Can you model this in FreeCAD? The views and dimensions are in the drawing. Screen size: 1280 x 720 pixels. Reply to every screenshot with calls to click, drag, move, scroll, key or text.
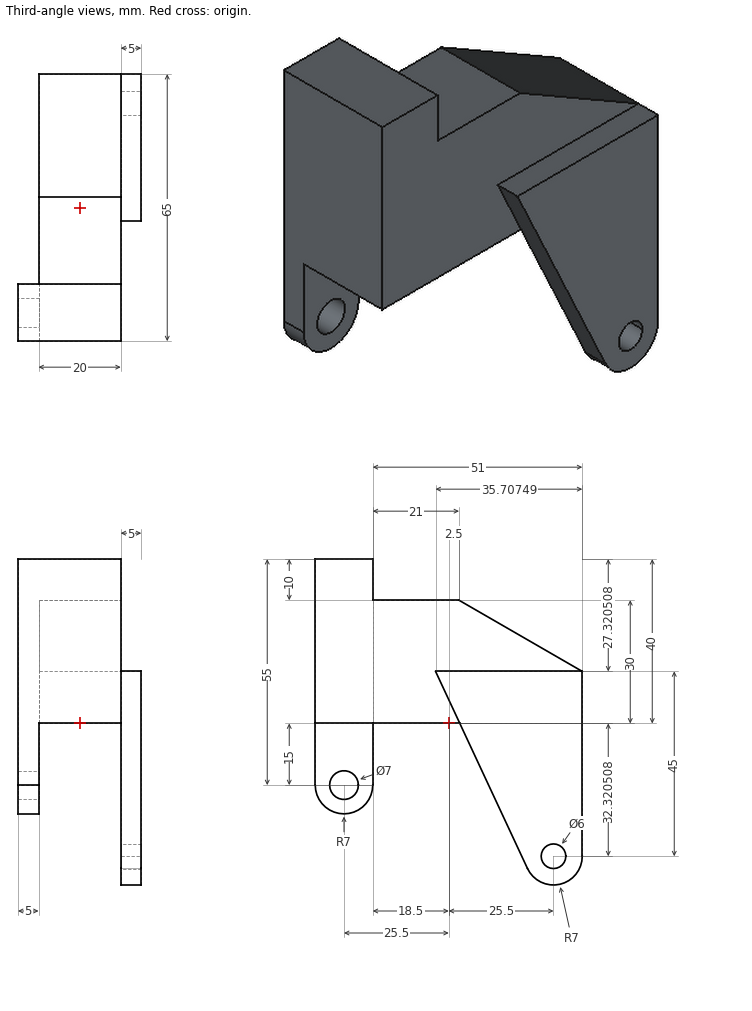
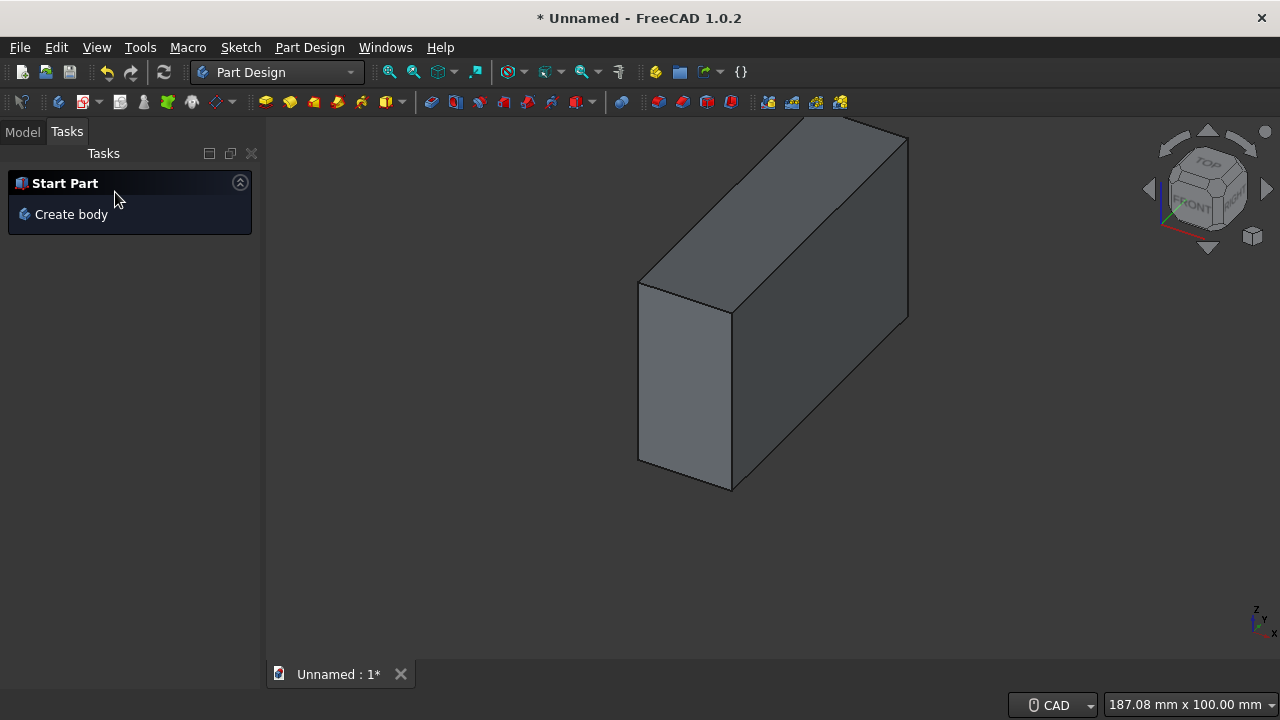
key(v)
key(f)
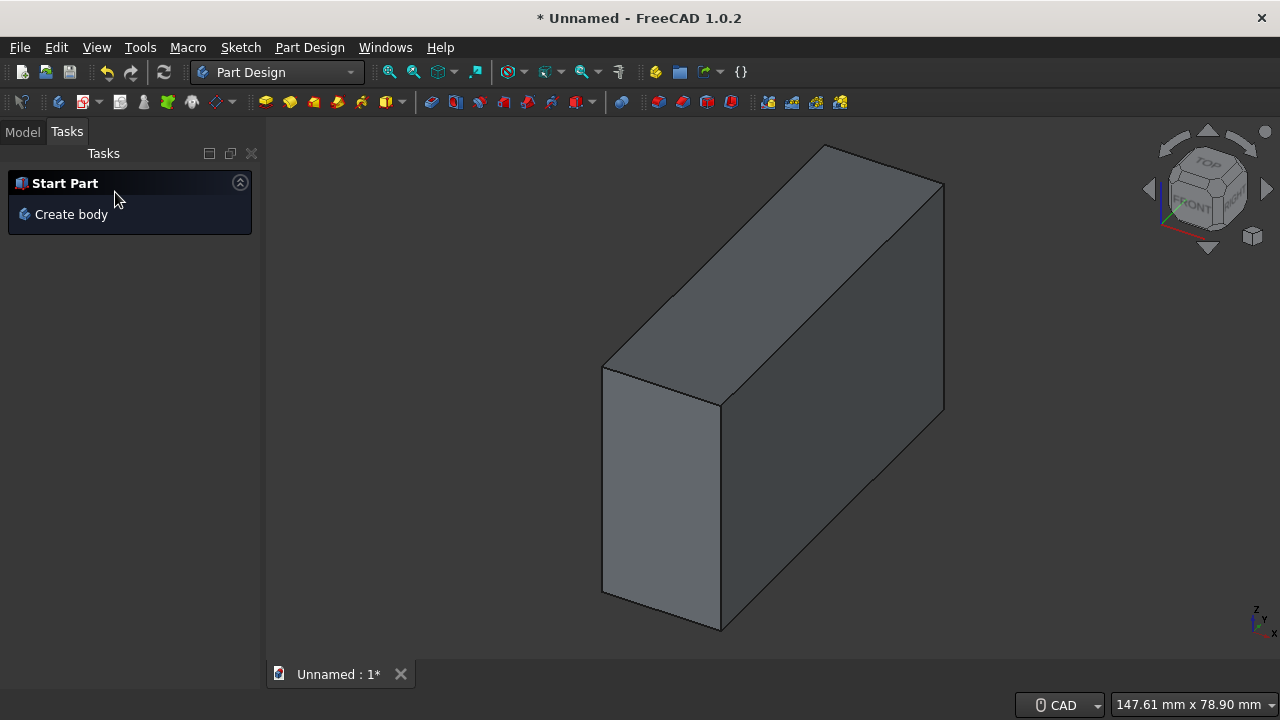
click(864, 375)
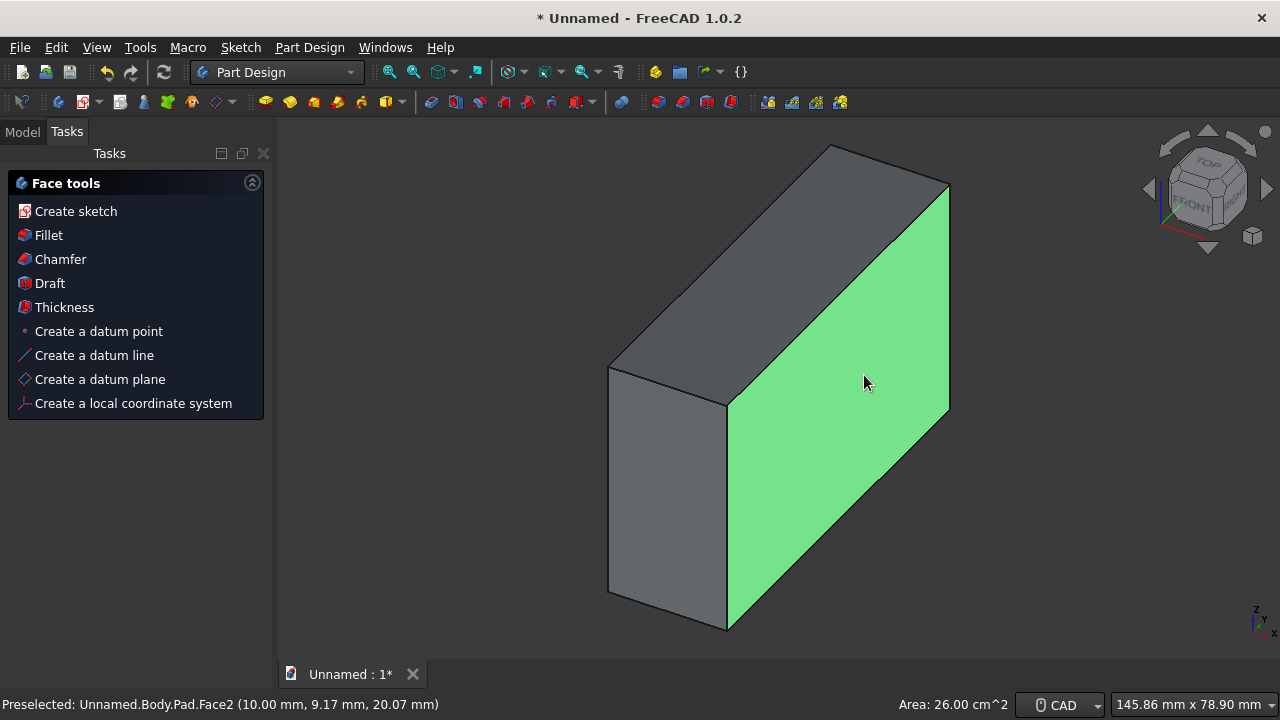
click(84, 102)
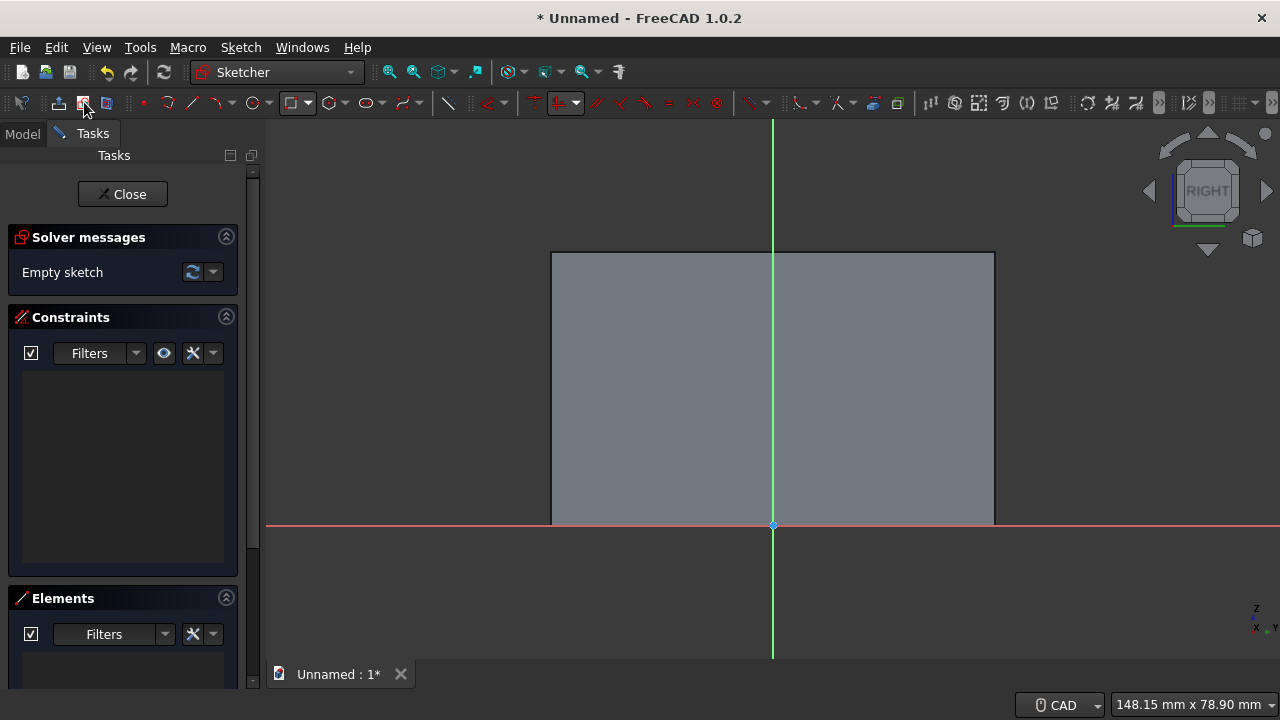
click(168, 104)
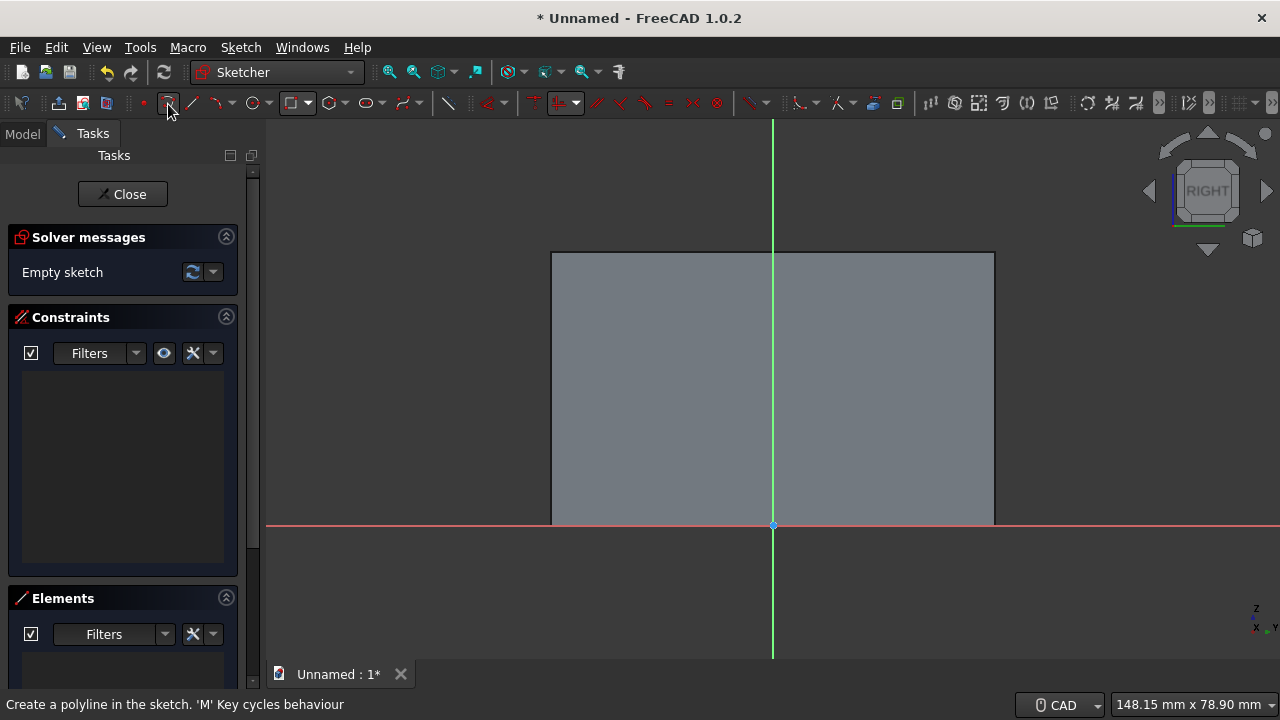
click(790, 321)
click(995, 439)
click(995, 252)
click(646, 252)
click(646, 321)
click(790, 322)
key(Escape)
key(Escape)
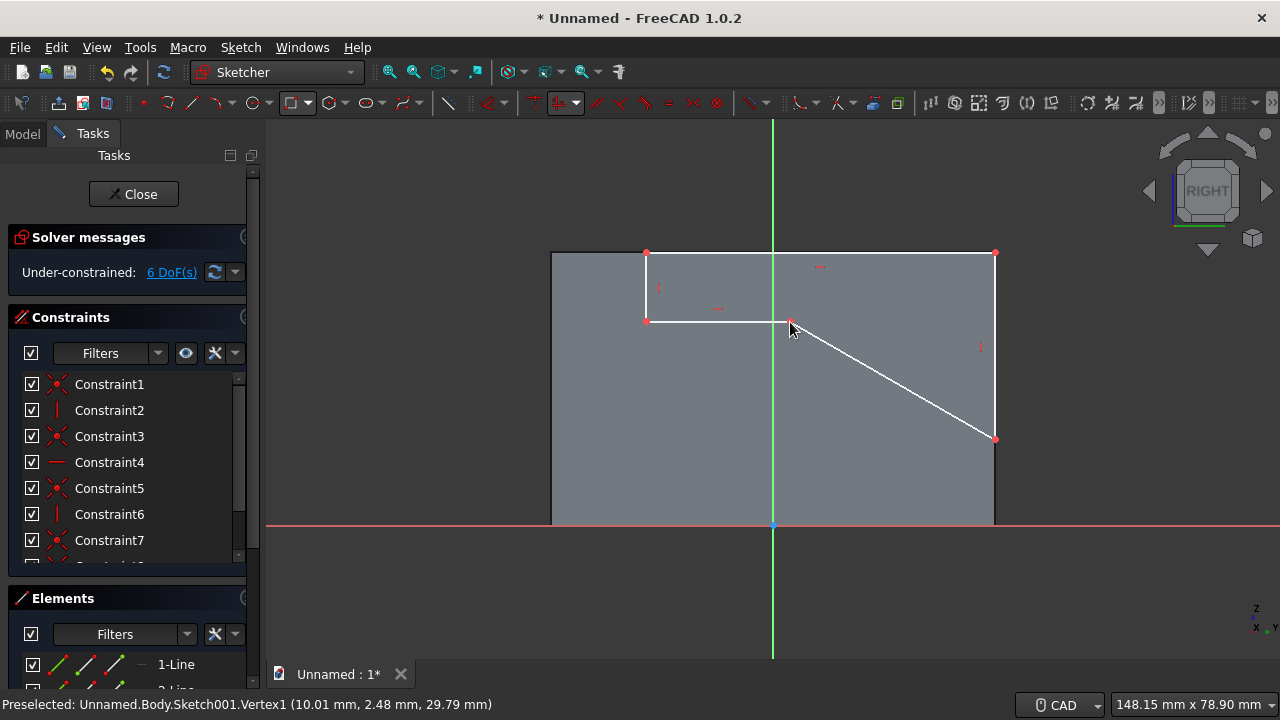
key(d)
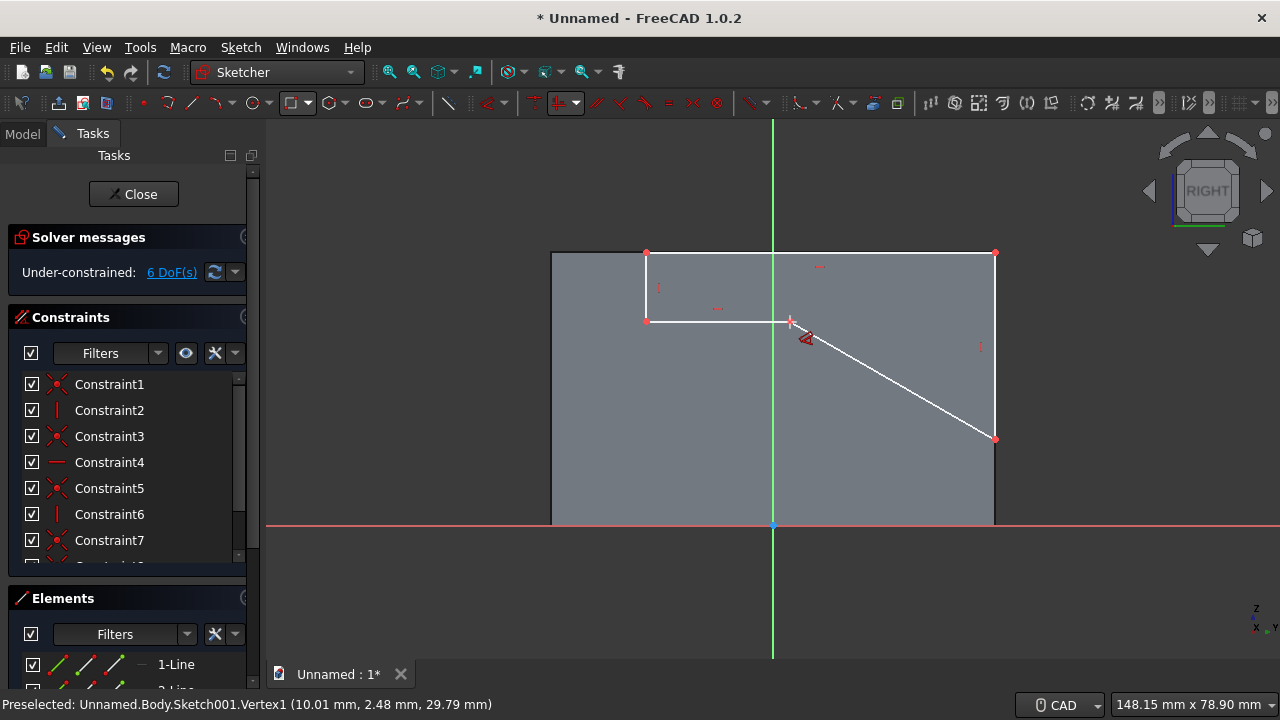
click(890, 253)
click(820, 219)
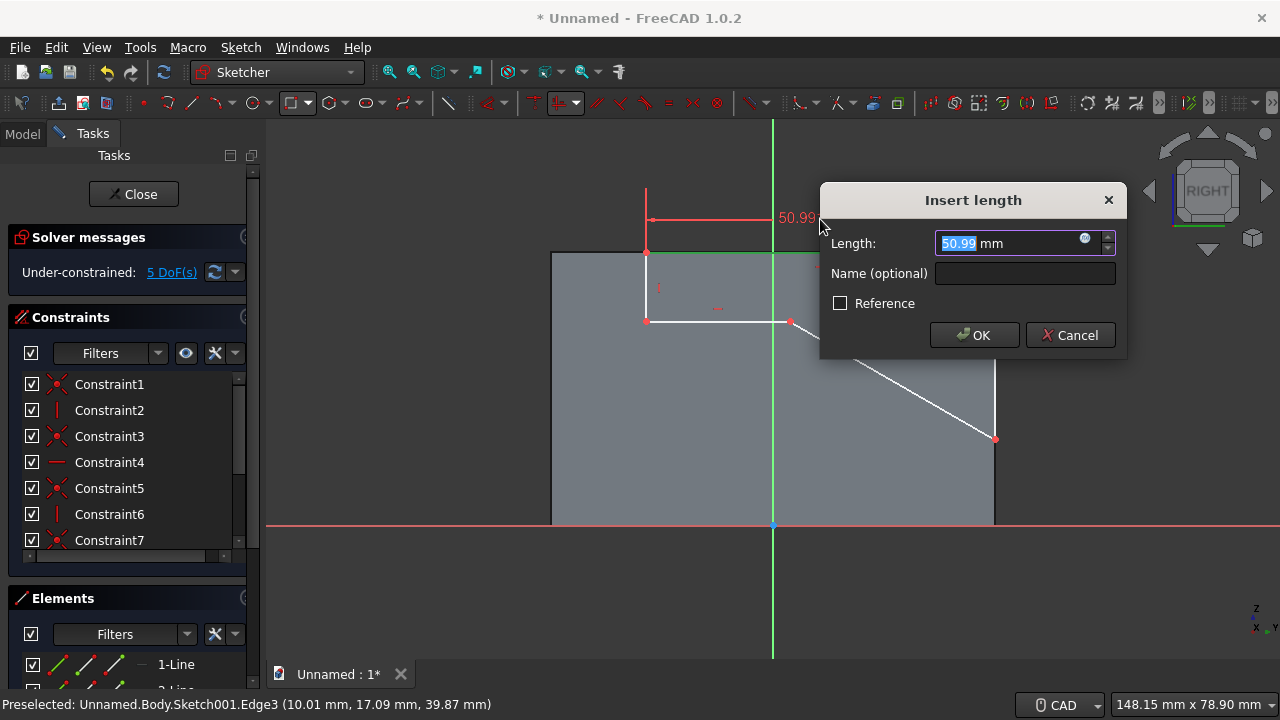
text(51)
key(Return)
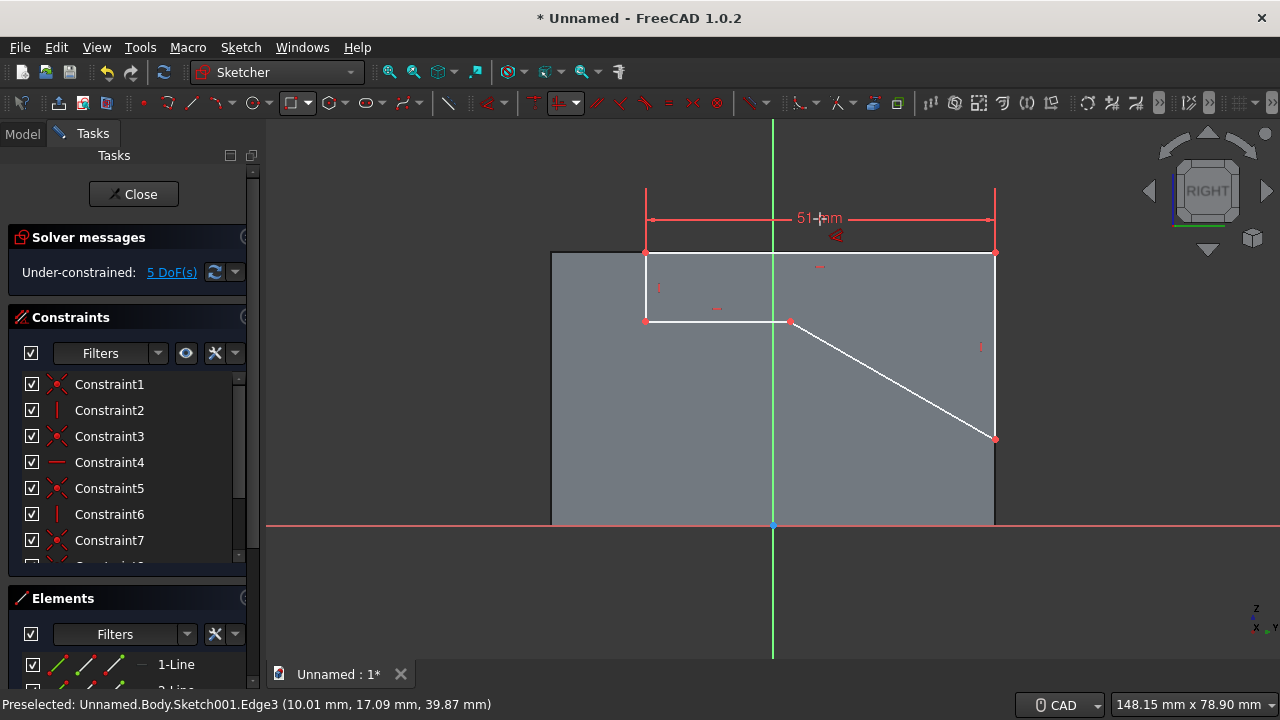
click(646, 274)
click(612, 287)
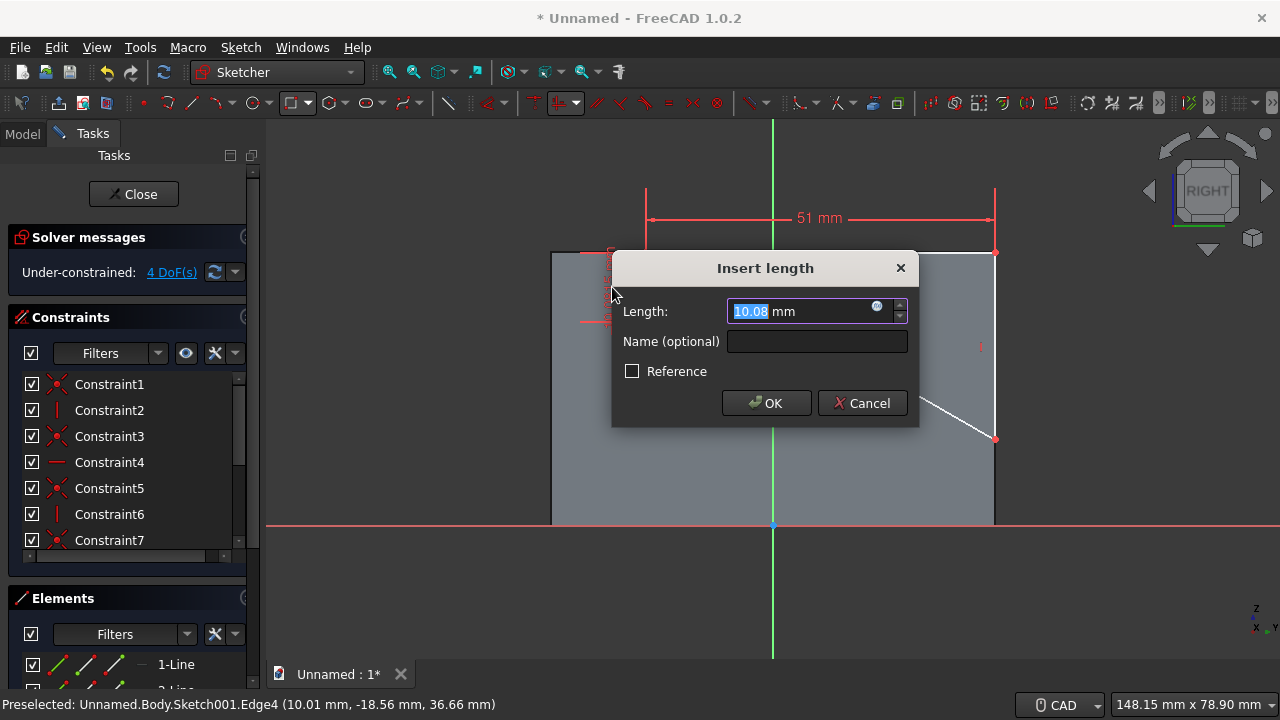
text(10)
key(Return)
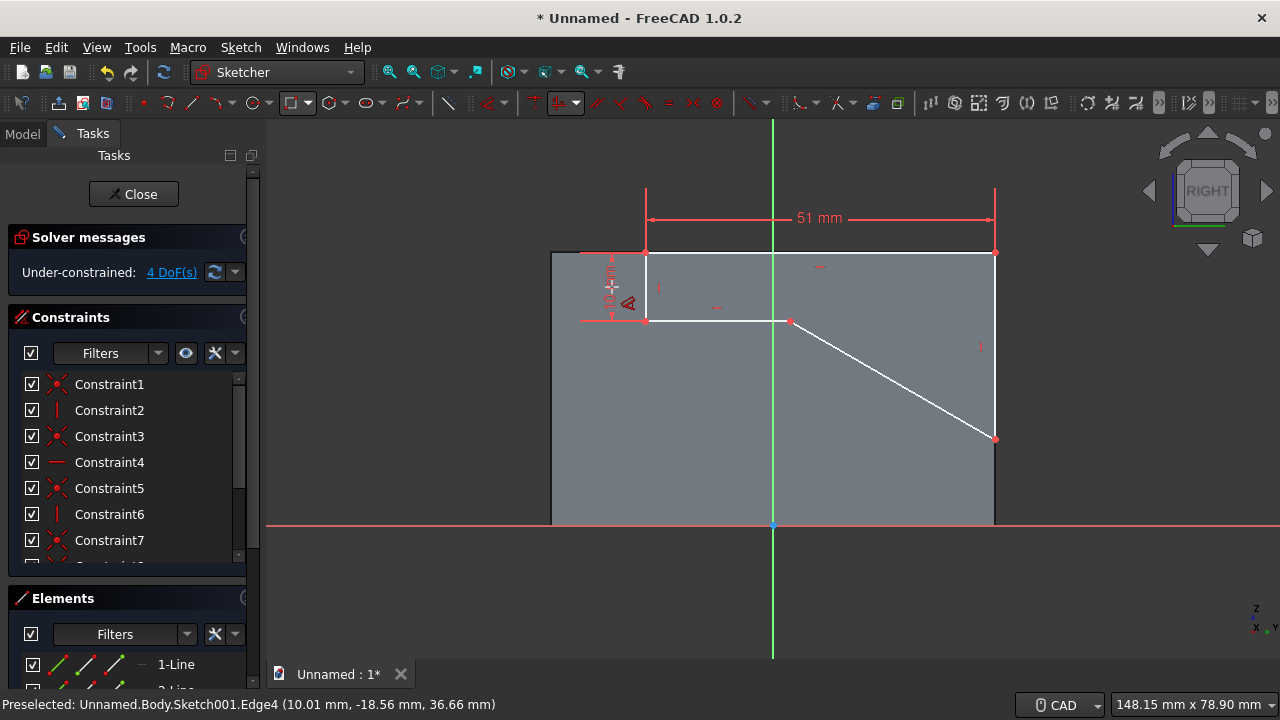
click(689, 321)
click(718, 287)